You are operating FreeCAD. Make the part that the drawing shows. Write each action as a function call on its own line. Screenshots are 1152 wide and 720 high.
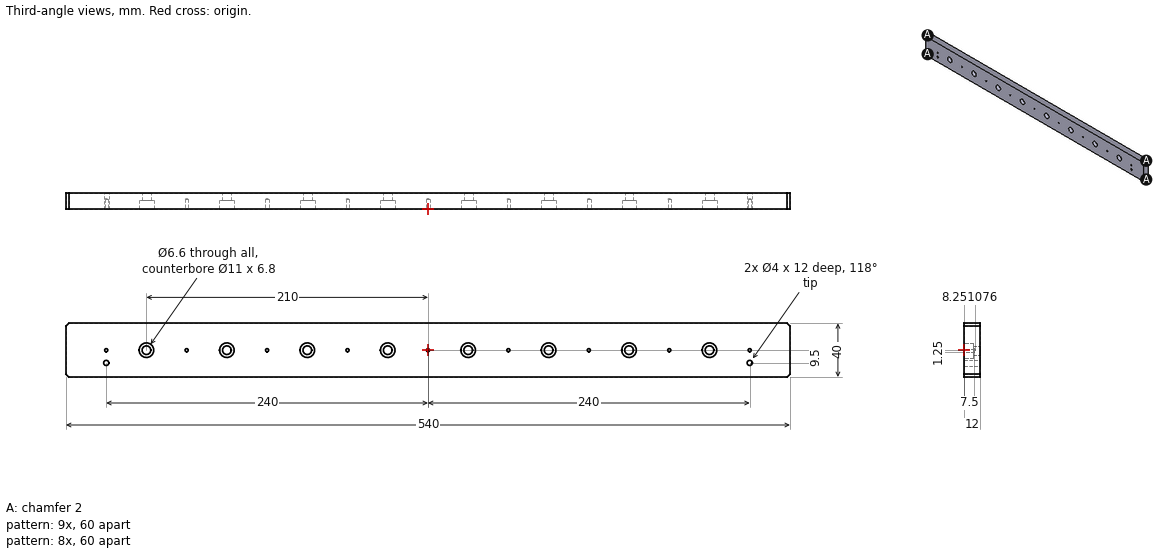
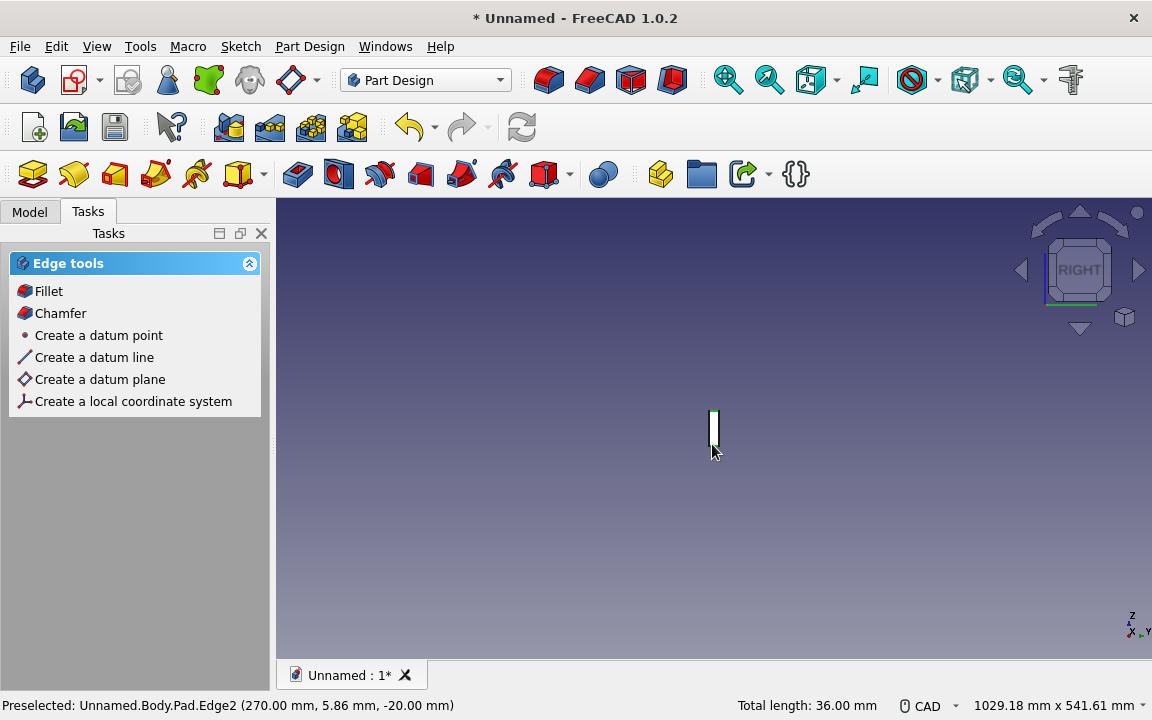
key(5)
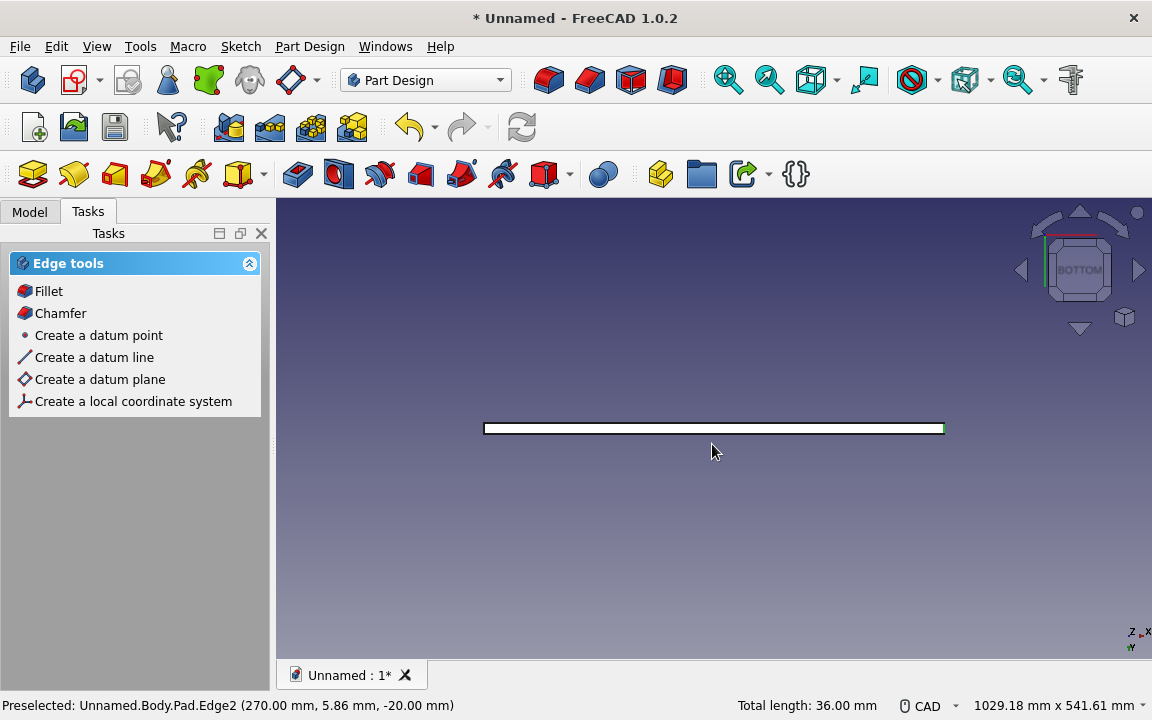
click(484, 429, ctrl)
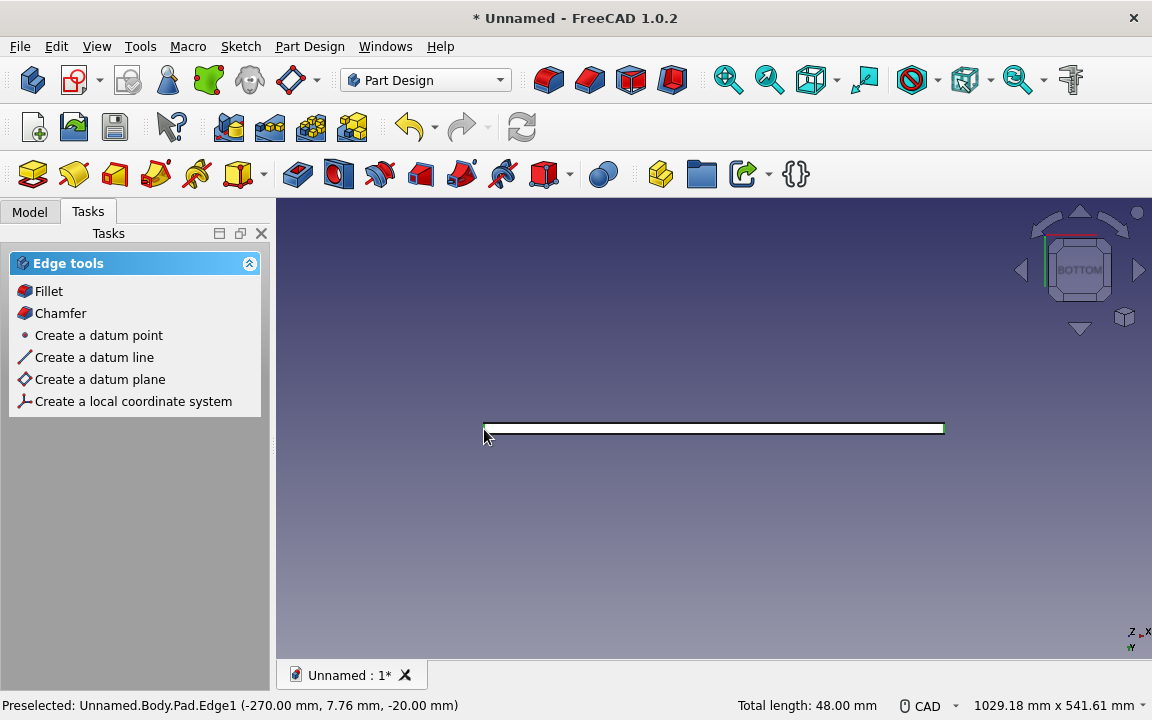
click(590, 80)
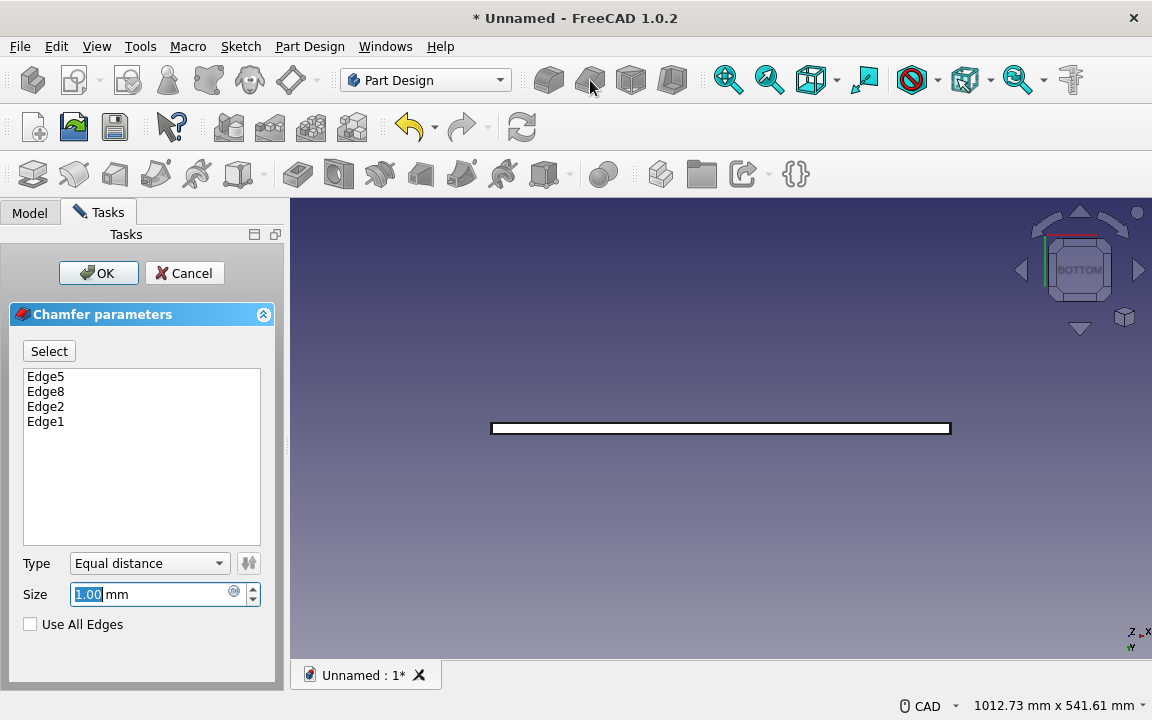
text(2)
key(Tab)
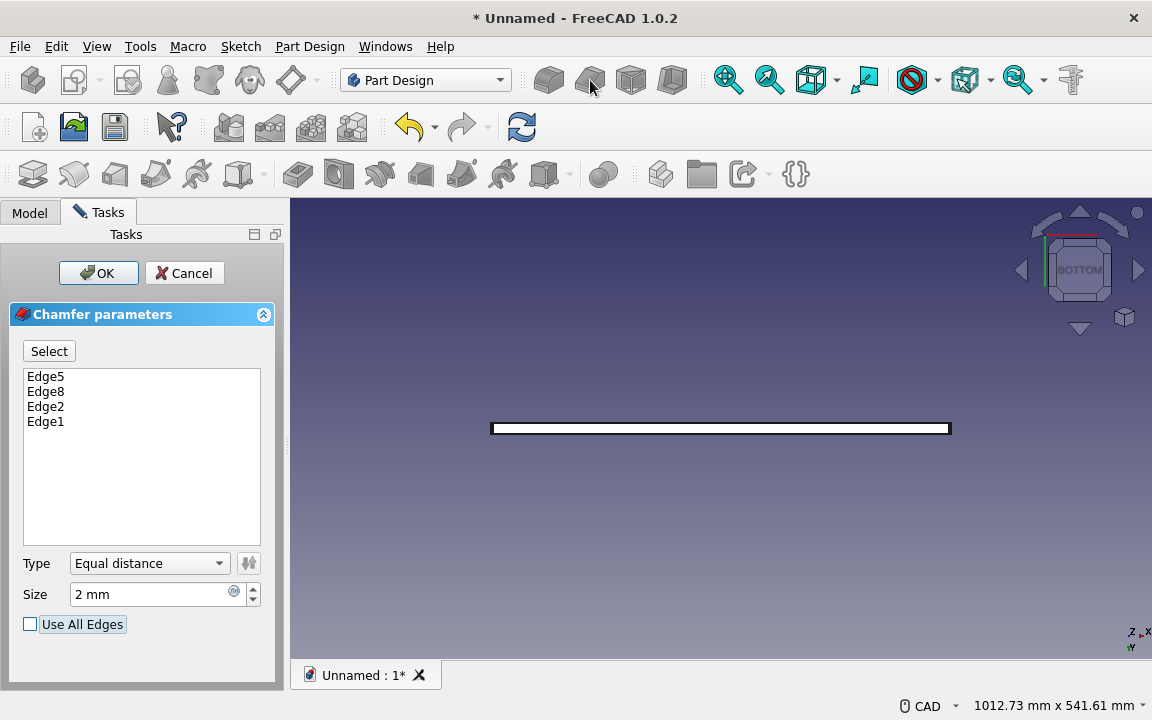
click(99, 273)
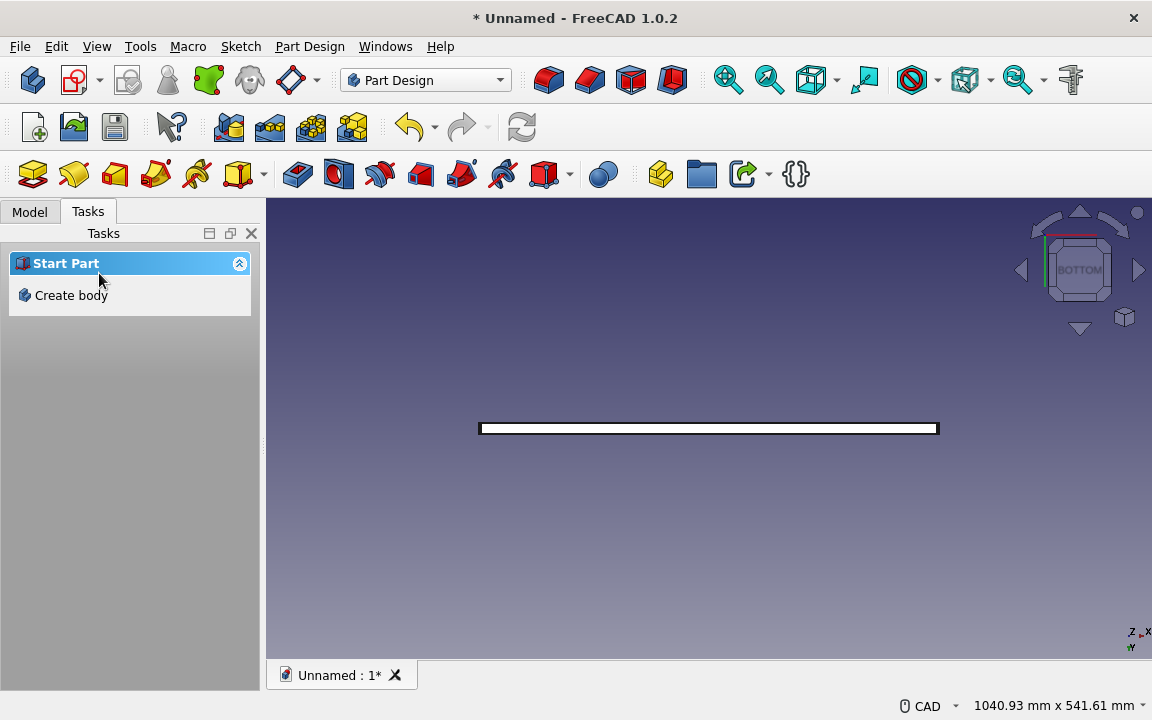
click(74, 80)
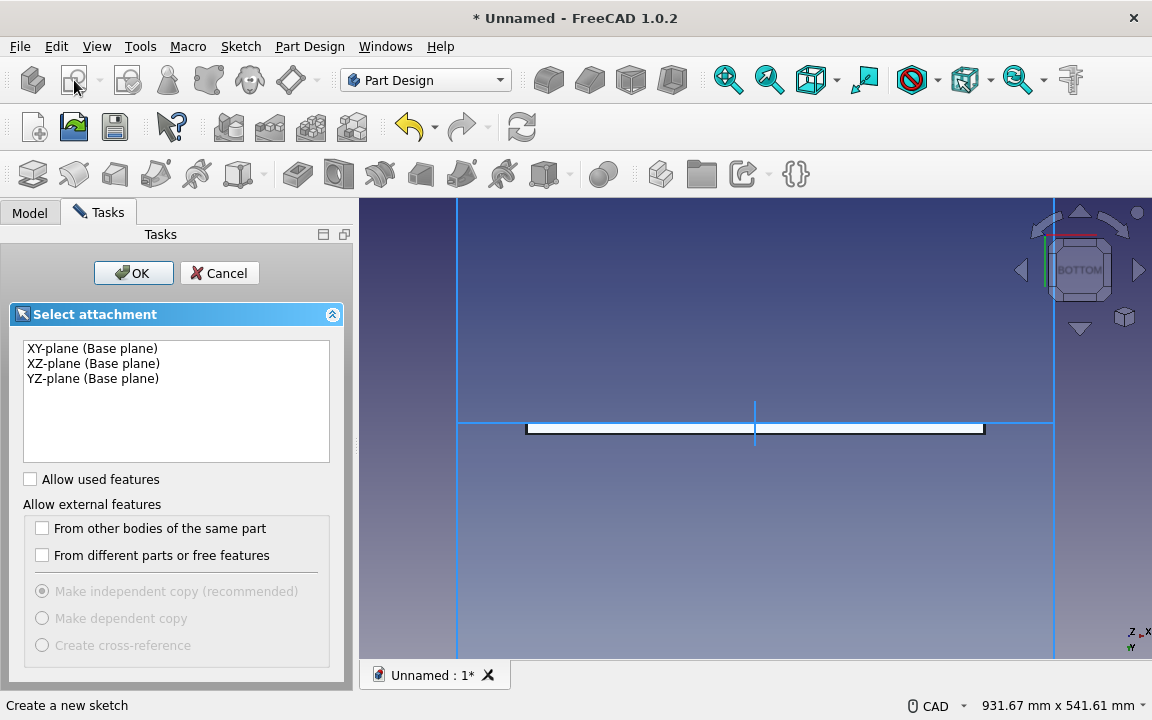
click(84, 364)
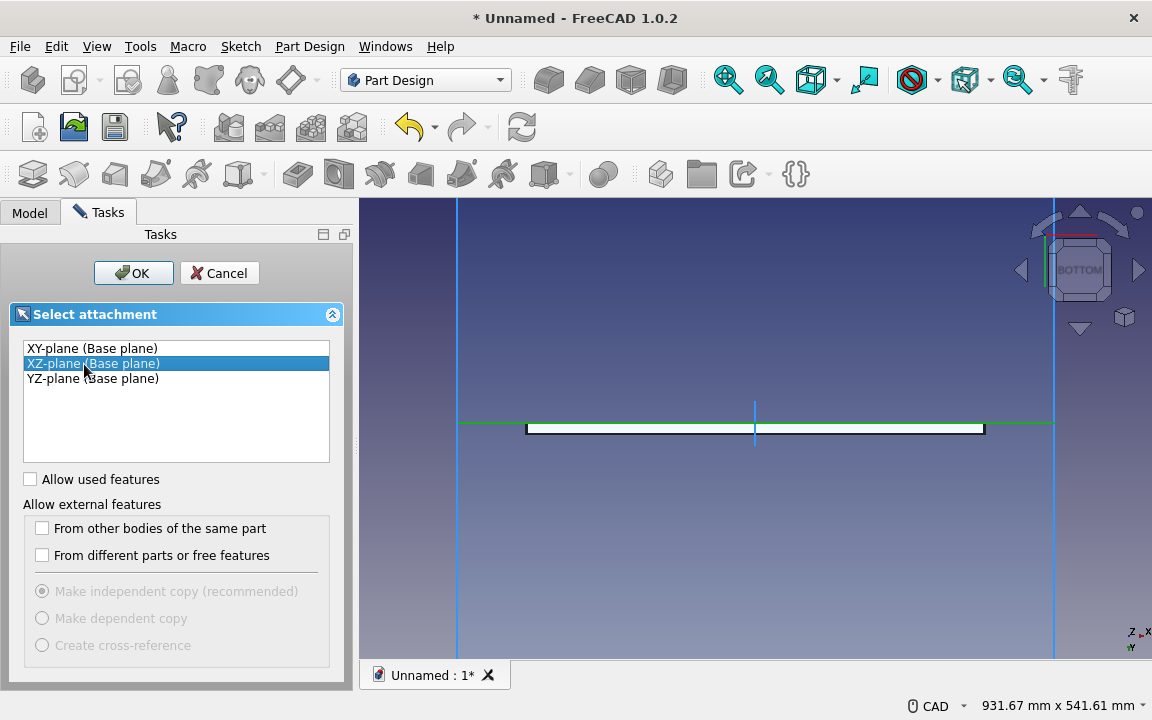
click(134, 273)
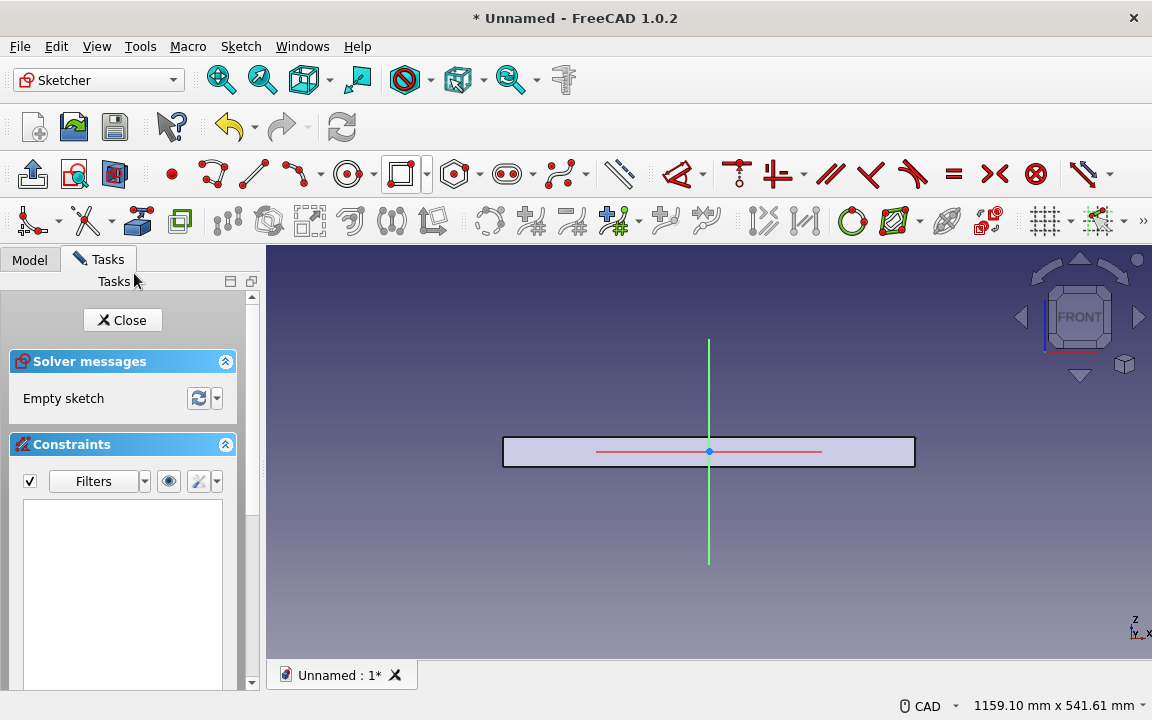
click(348, 174)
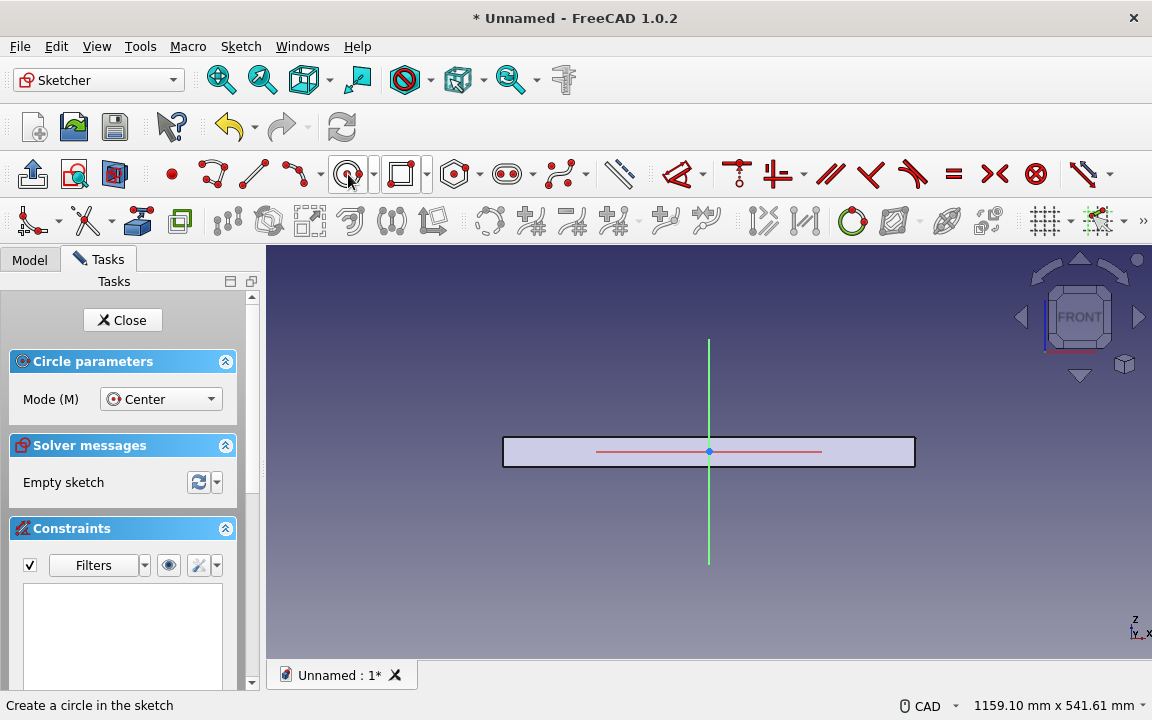
scroll(892, 459, up, 14)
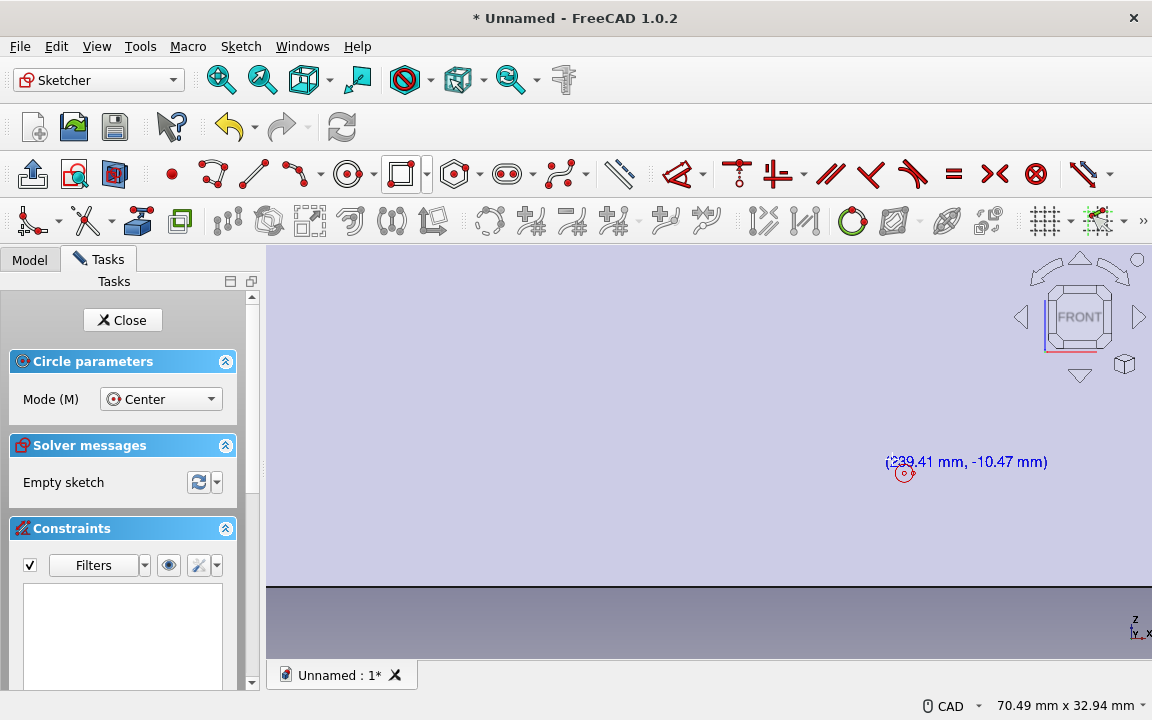
scroll(863, 456, down, 13)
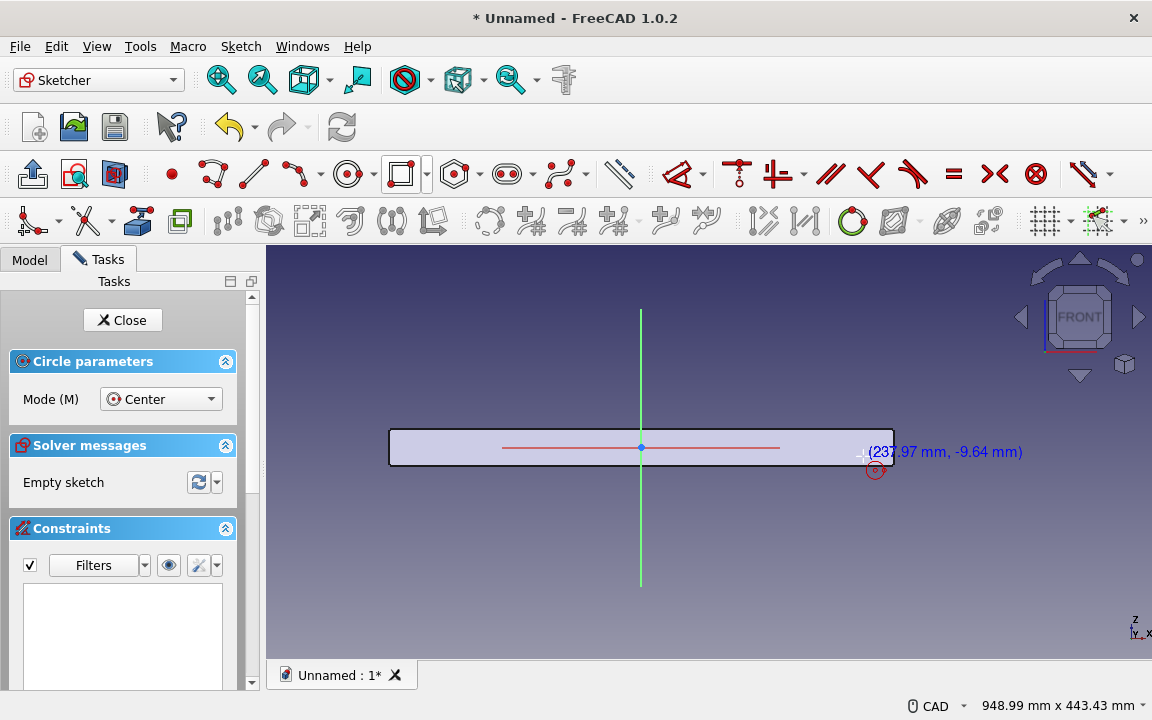
scroll(866, 456, up, 3)